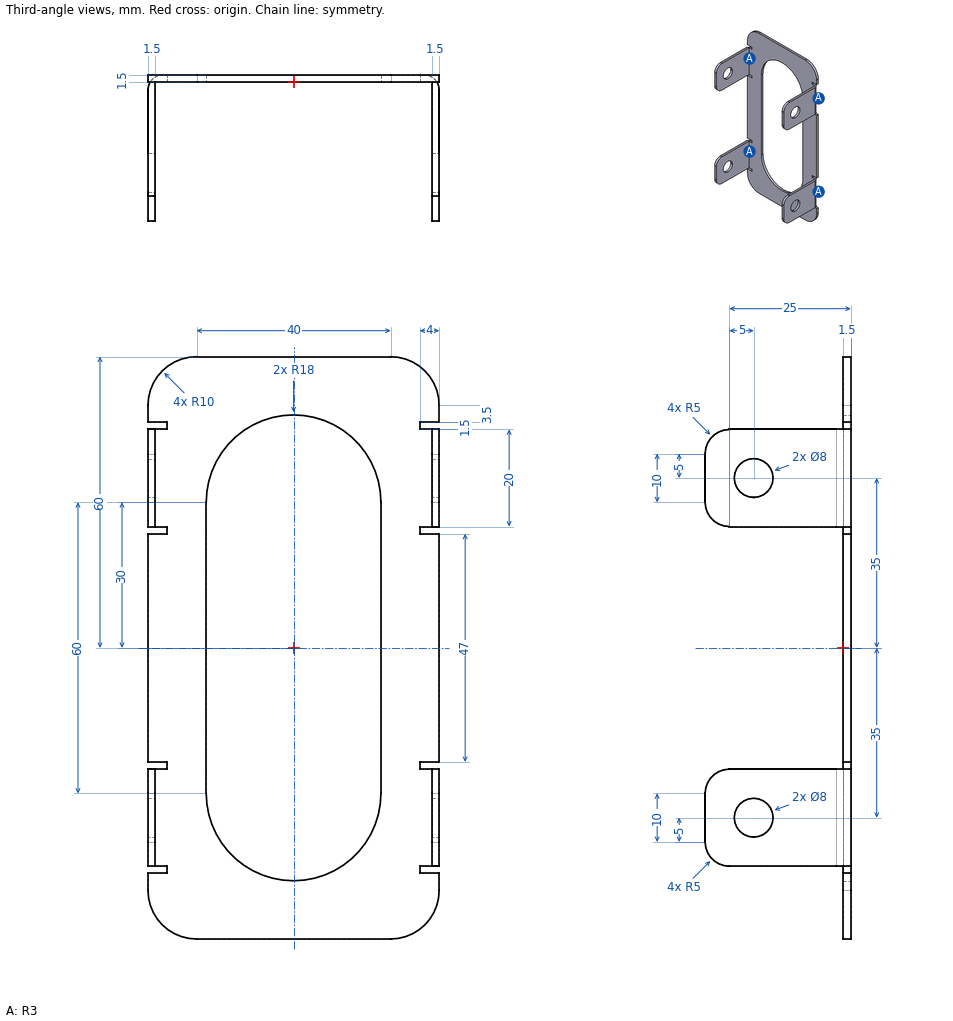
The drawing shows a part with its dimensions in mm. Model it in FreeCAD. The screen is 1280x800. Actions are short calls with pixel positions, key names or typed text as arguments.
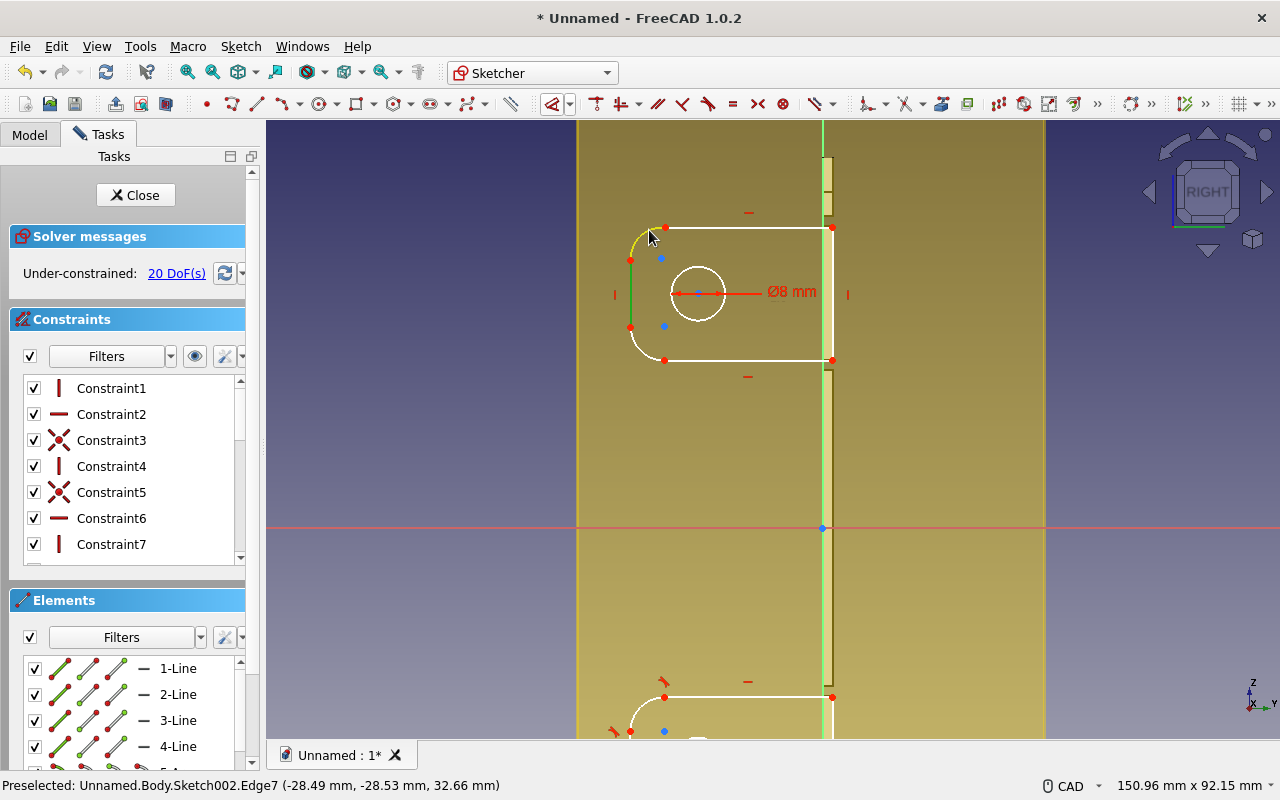
click(649, 230)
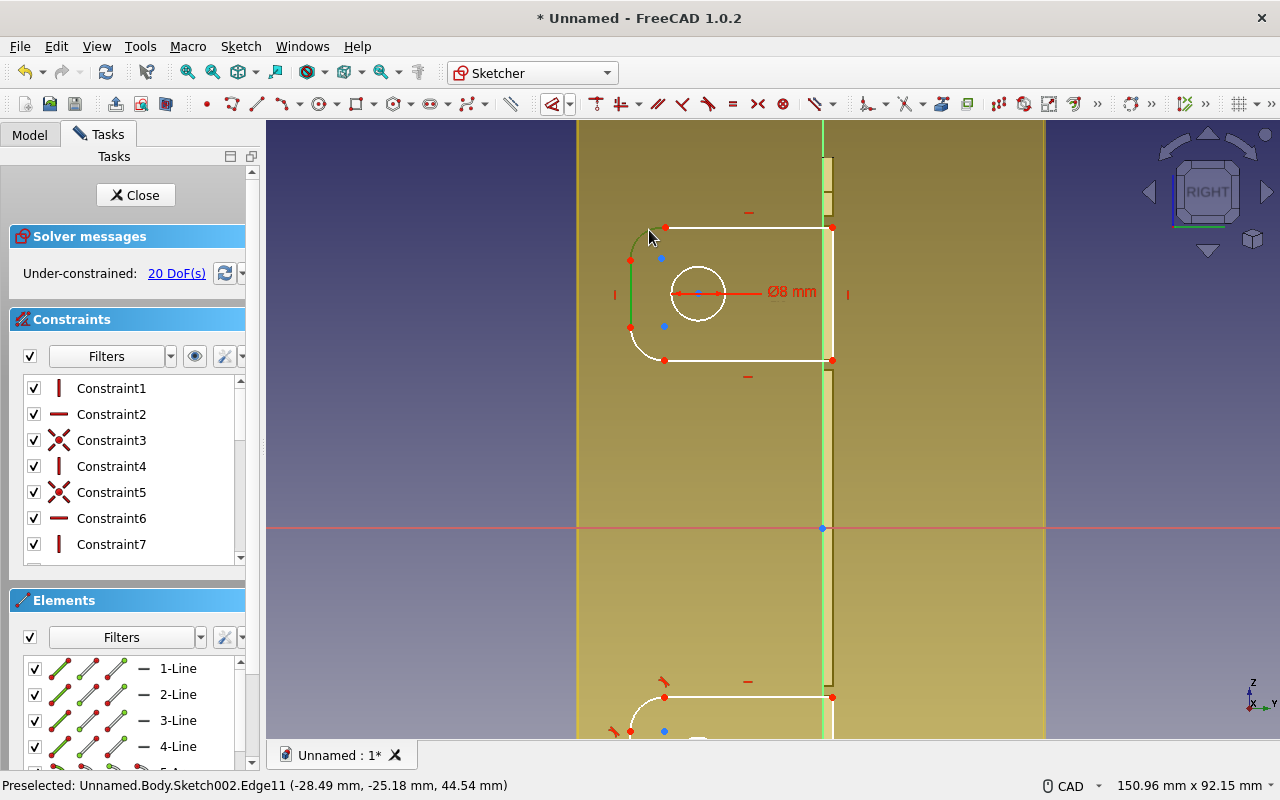
key(t)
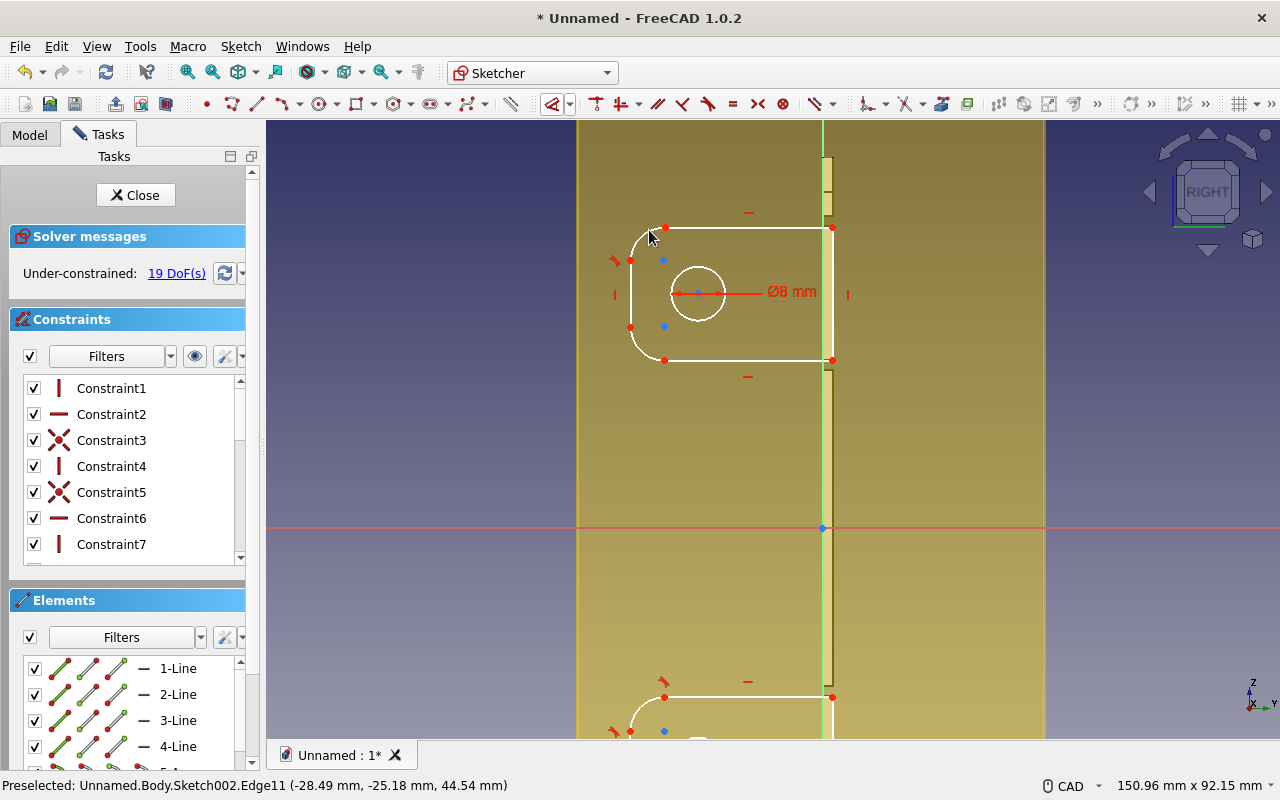
click(631, 308)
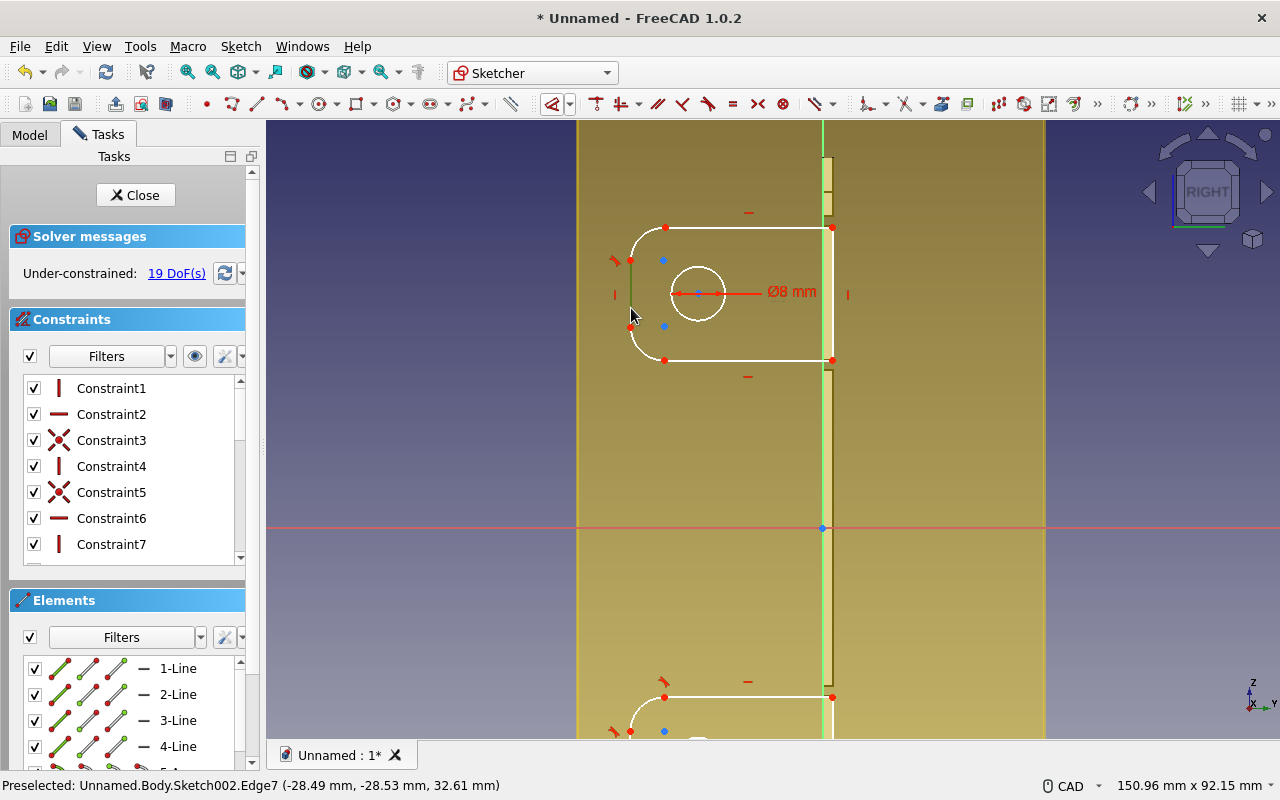
click(635, 343)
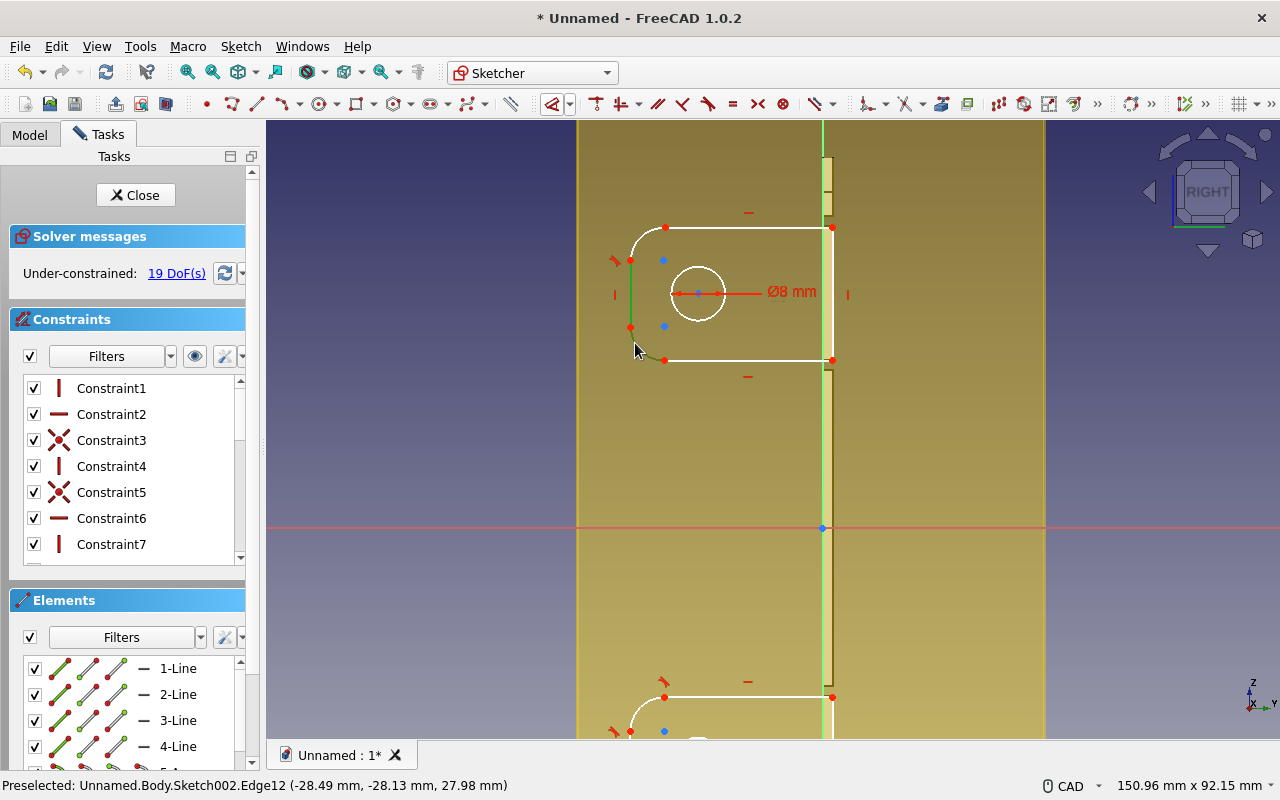
key(t)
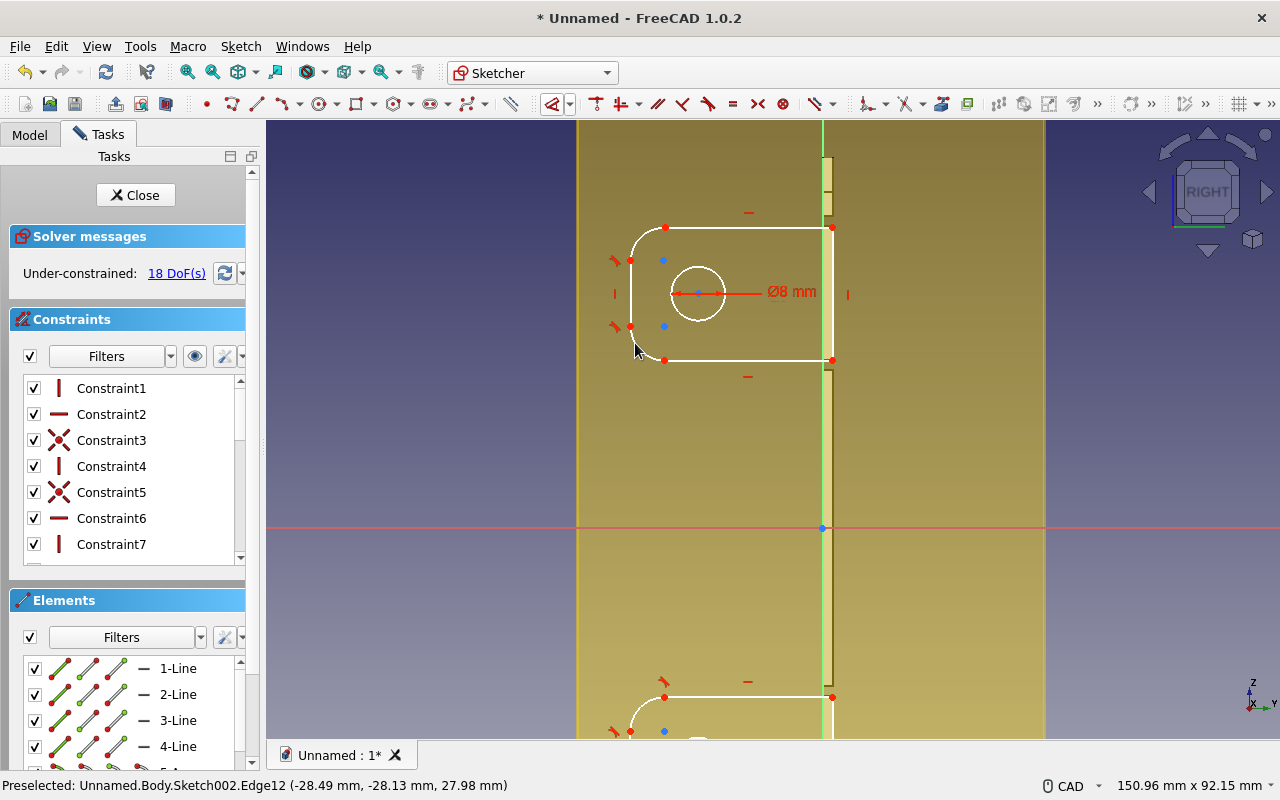
click(715, 228)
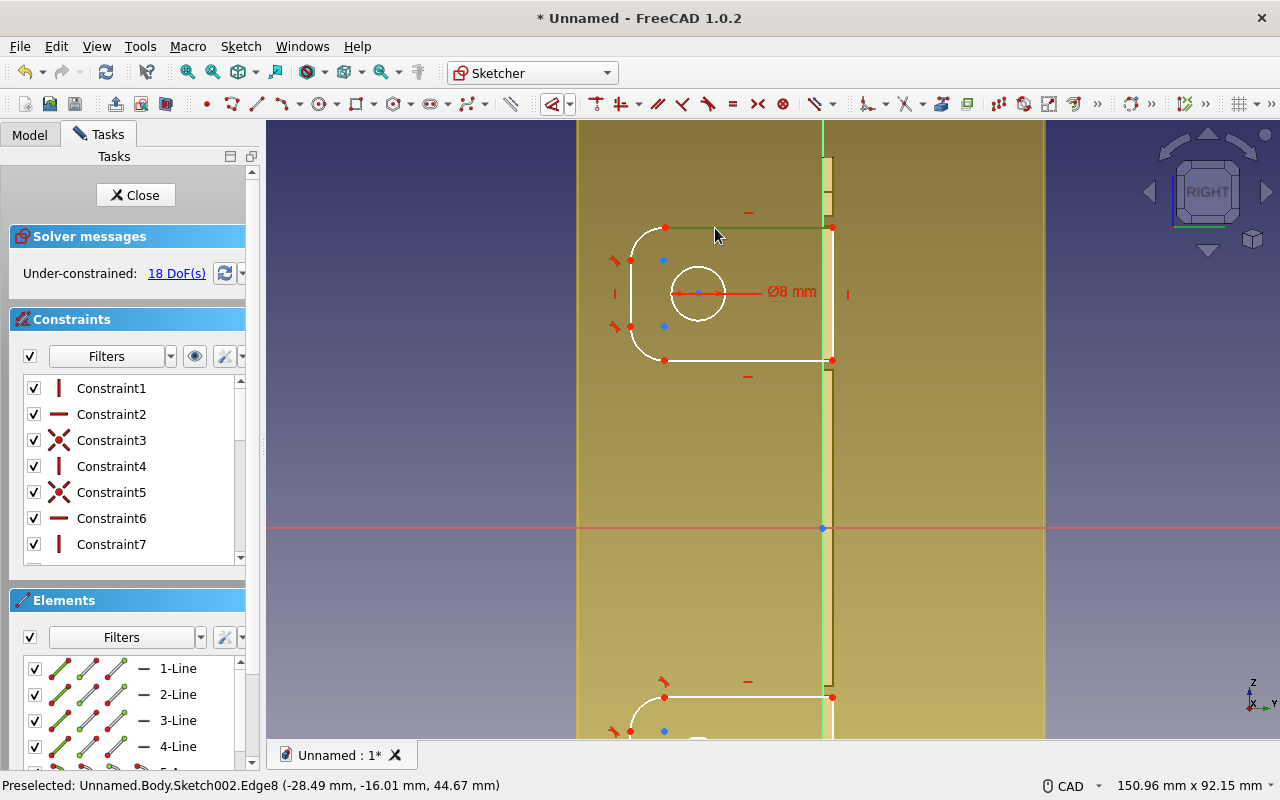
click(650, 231)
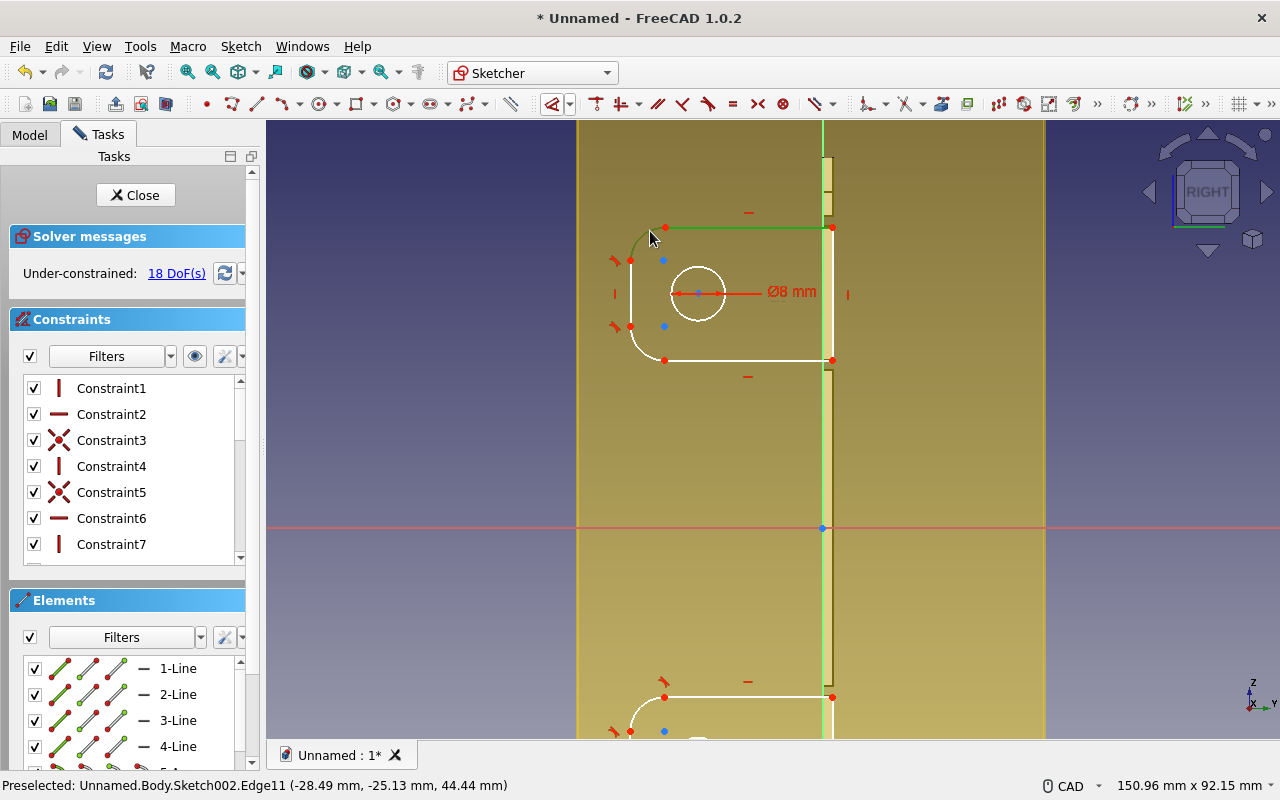
click(708, 104)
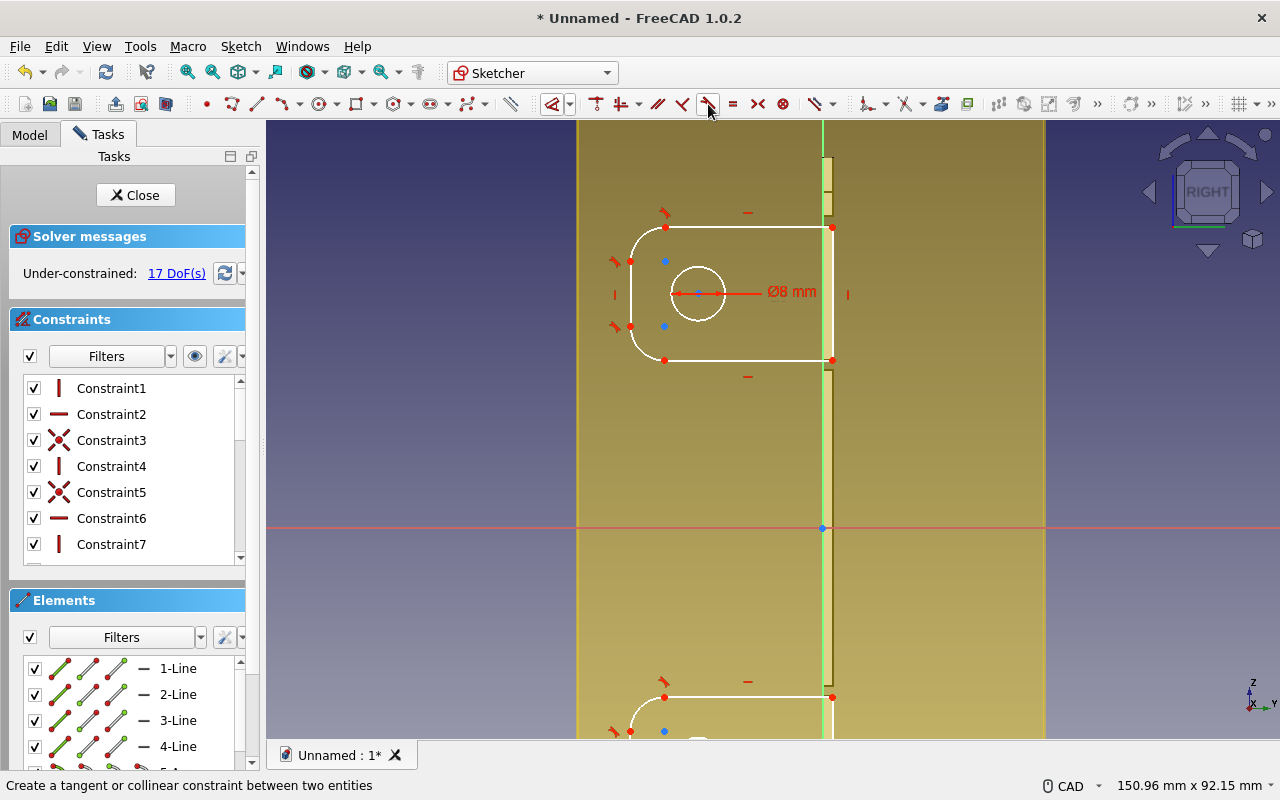
click(782, 361)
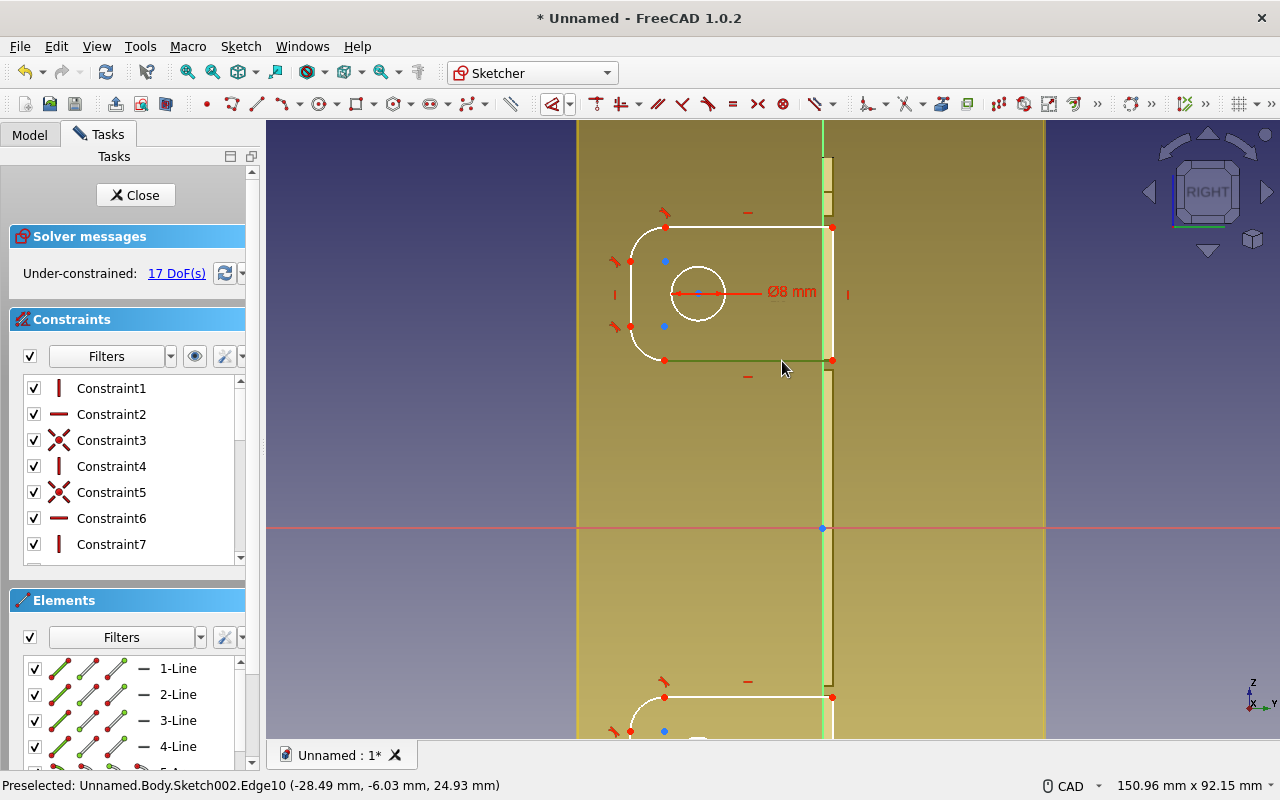
click(635, 342)